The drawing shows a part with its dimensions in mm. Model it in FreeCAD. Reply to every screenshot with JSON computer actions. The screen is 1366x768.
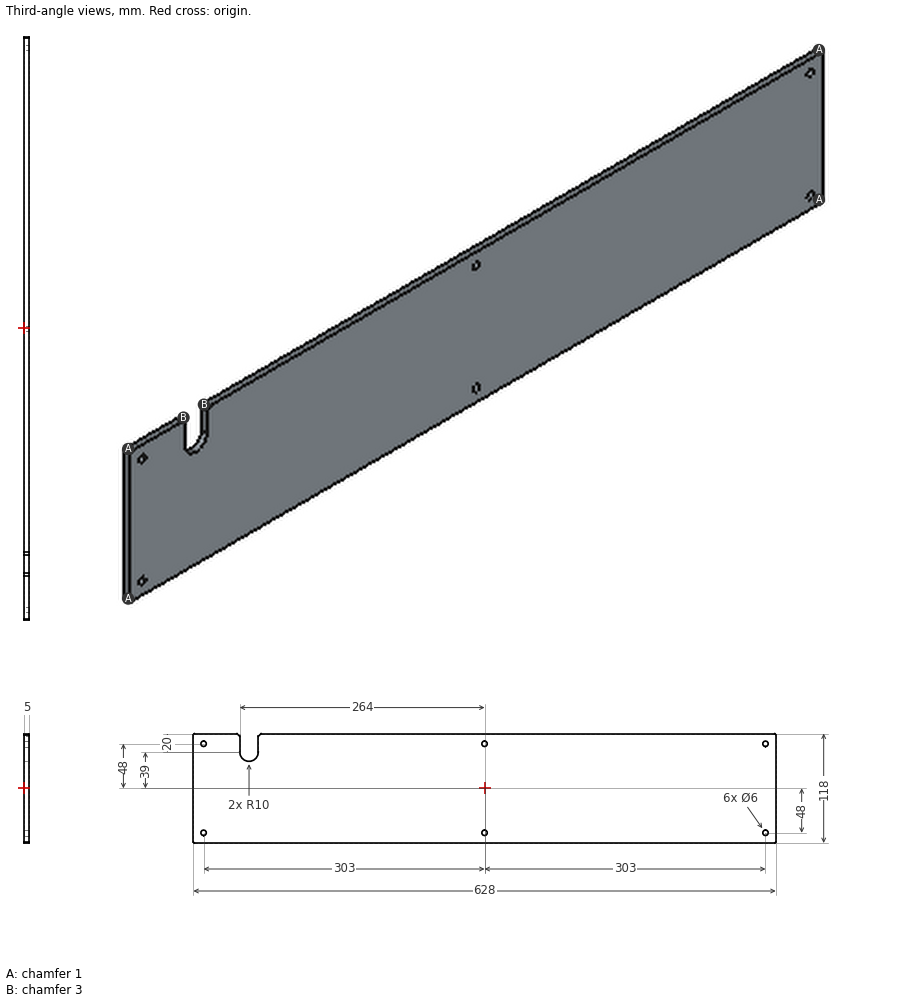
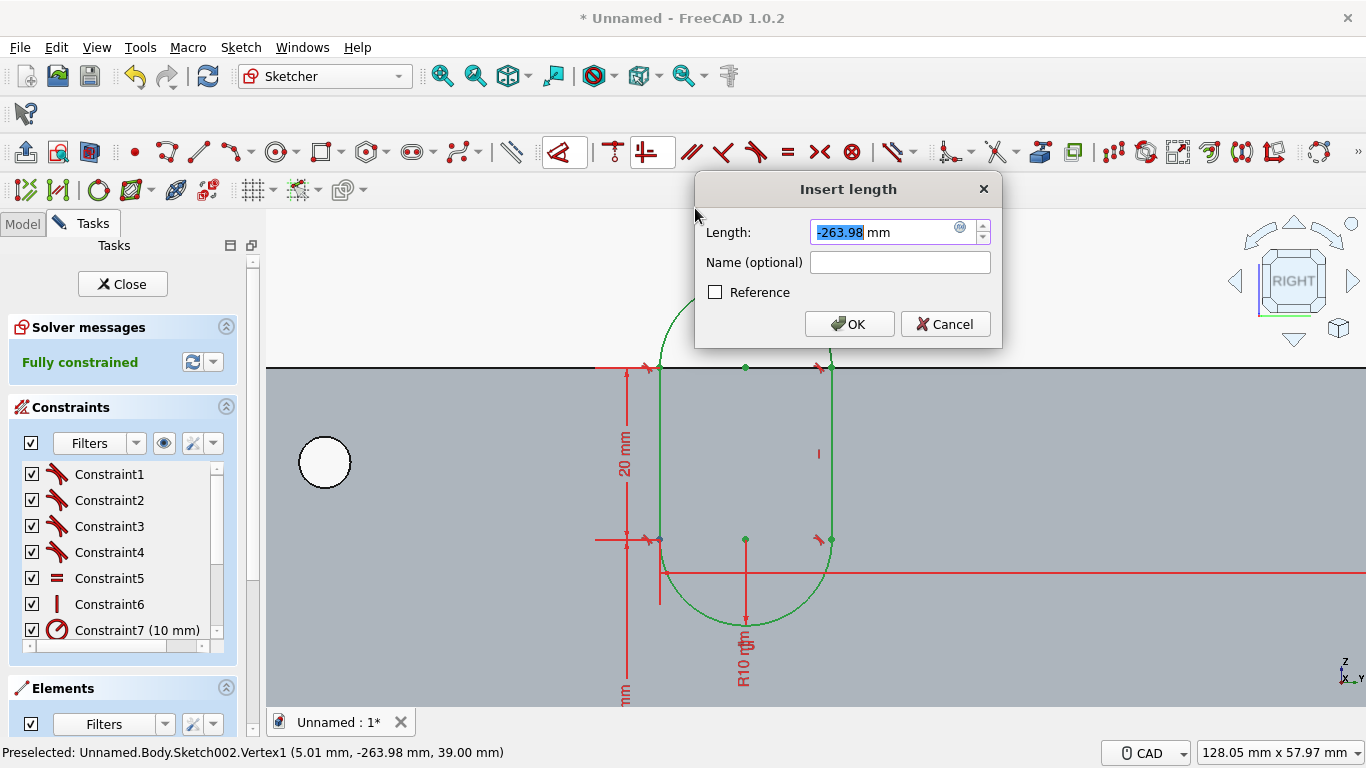
{"action": "type", "text": "-264"}
{"action": "key", "text": "Return"}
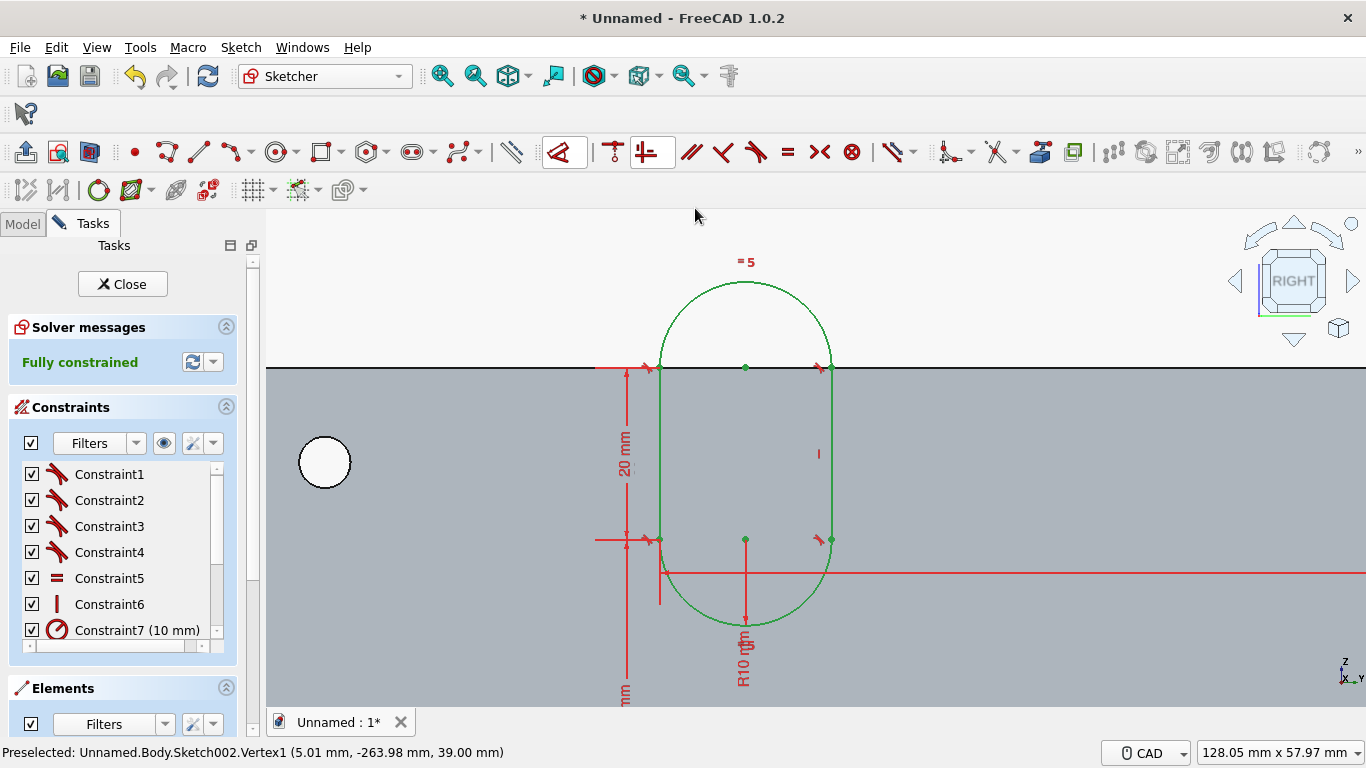
{"action": "left_click", "coordinate": [123, 284]}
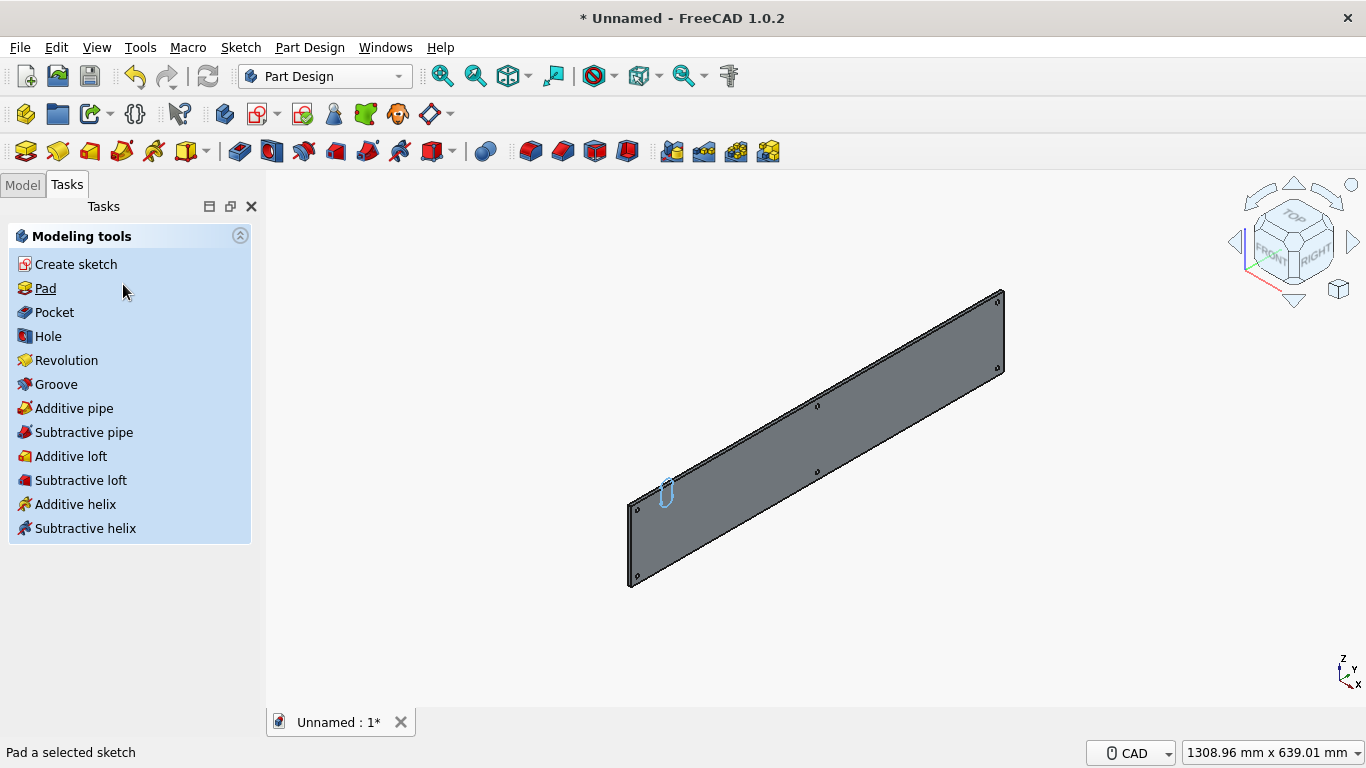
{"action": "left_click", "coordinate": [240, 152]}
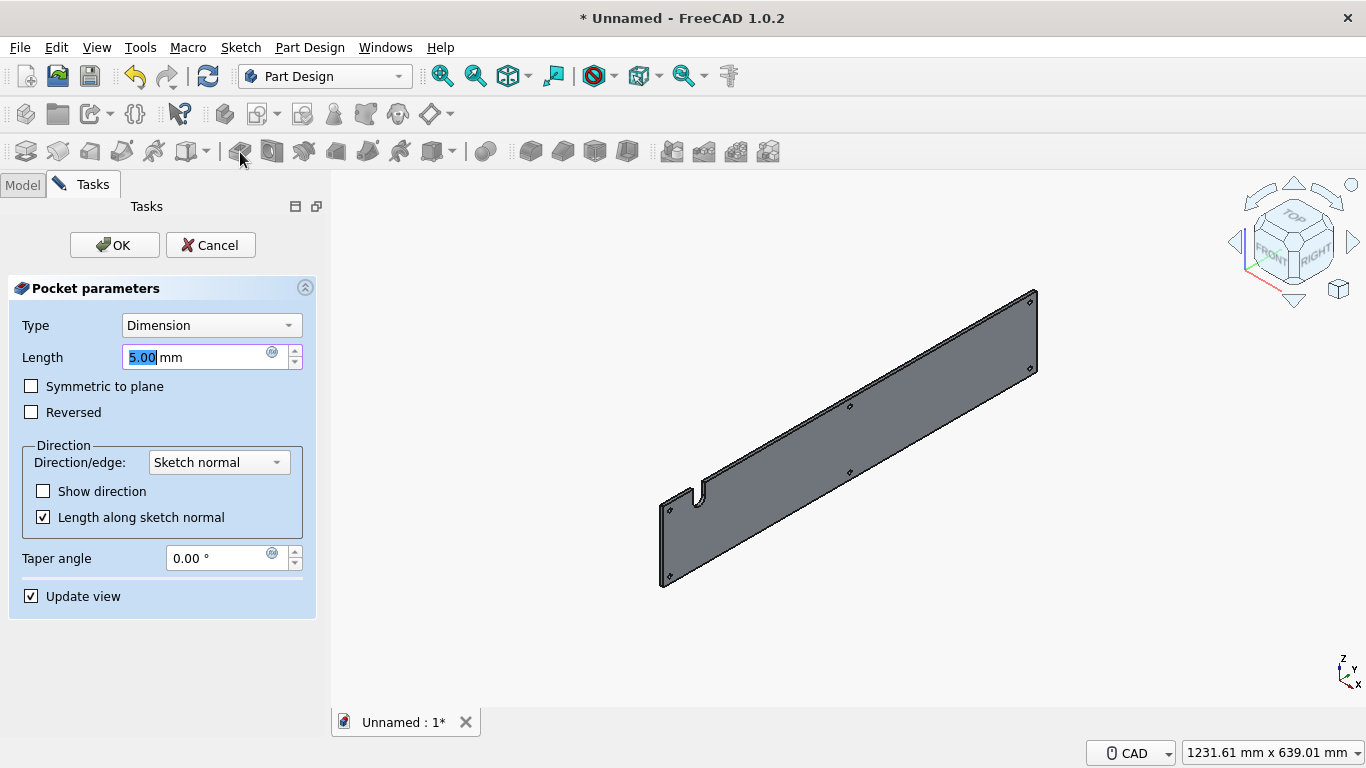
{"action": "left_click", "coordinate": [212, 326]}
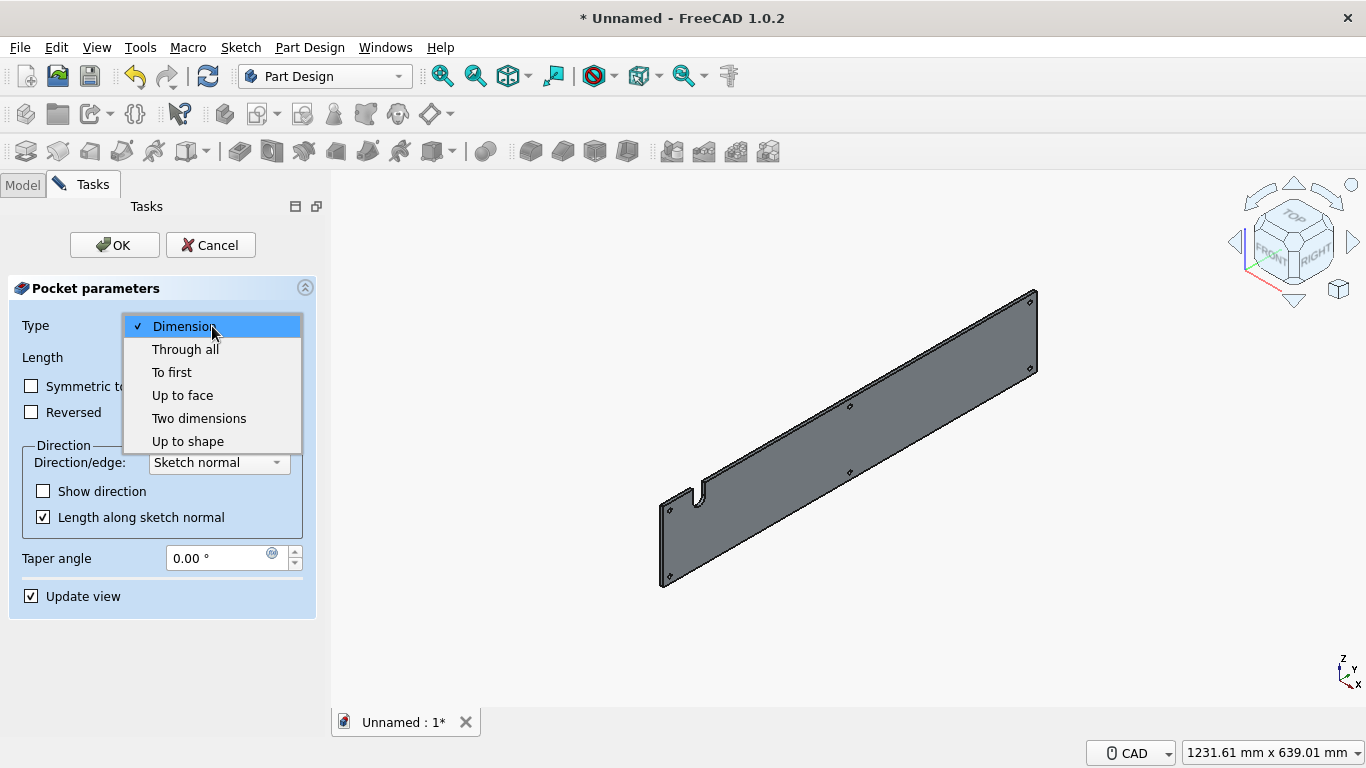
{"action": "left_click", "coordinate": [212, 350]}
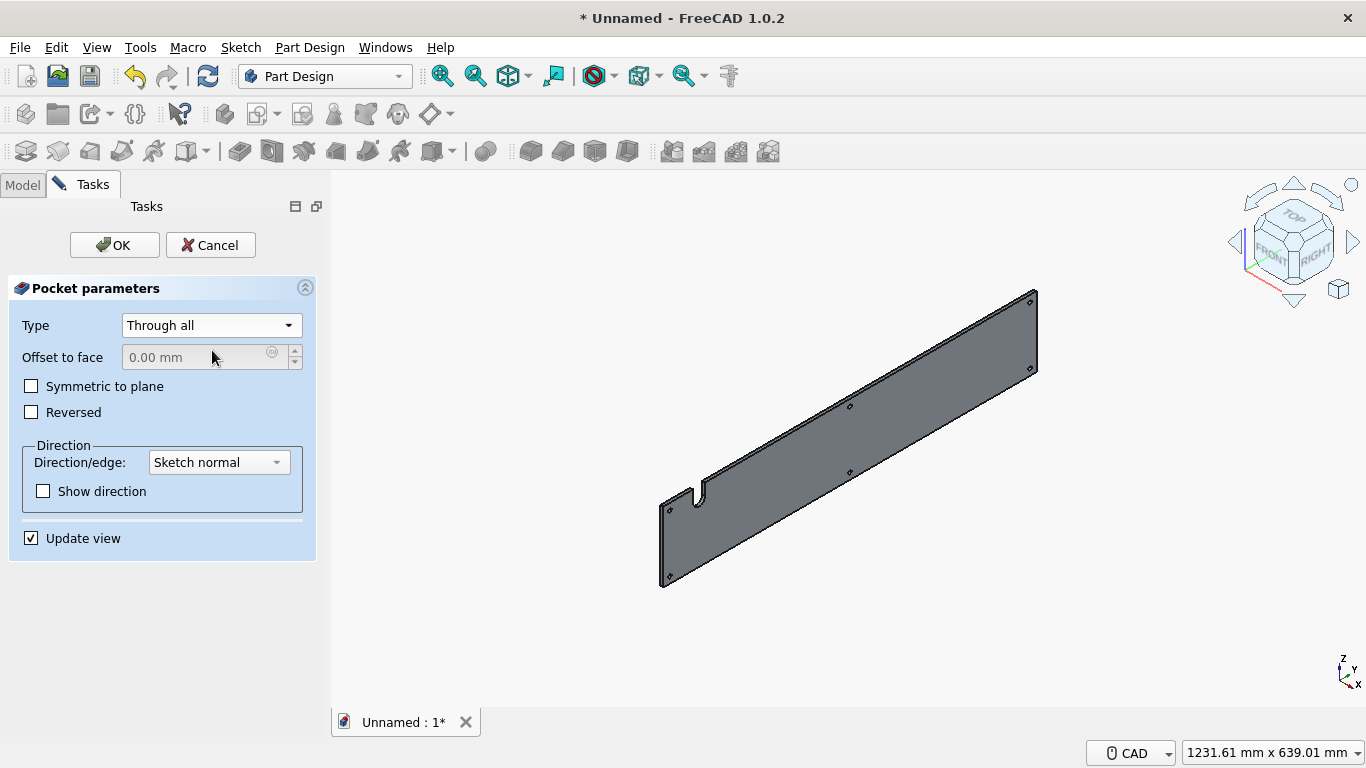
{"action": "left_click", "coordinate": [115, 245]}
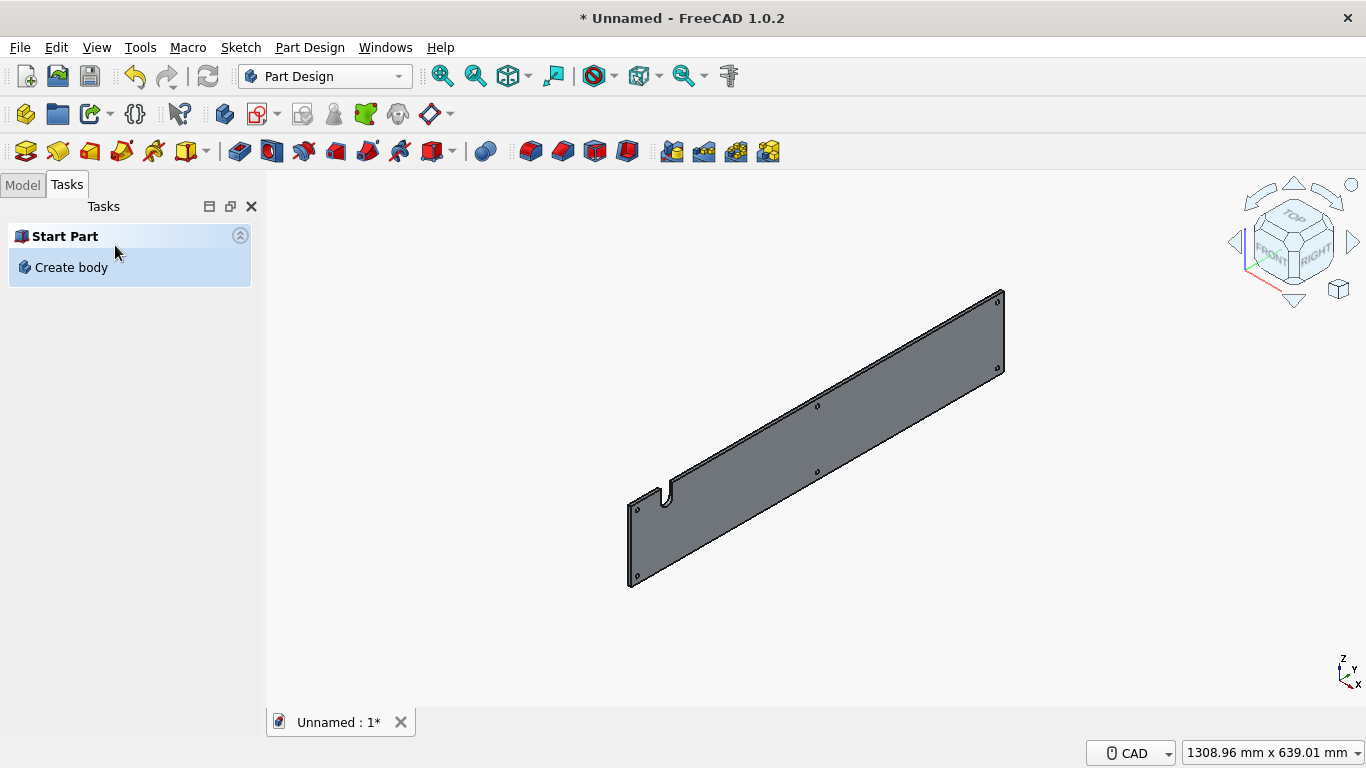
{"action": "scroll", "coordinate": [659, 488], "scroll_direction": "up", "scroll_amount": 12}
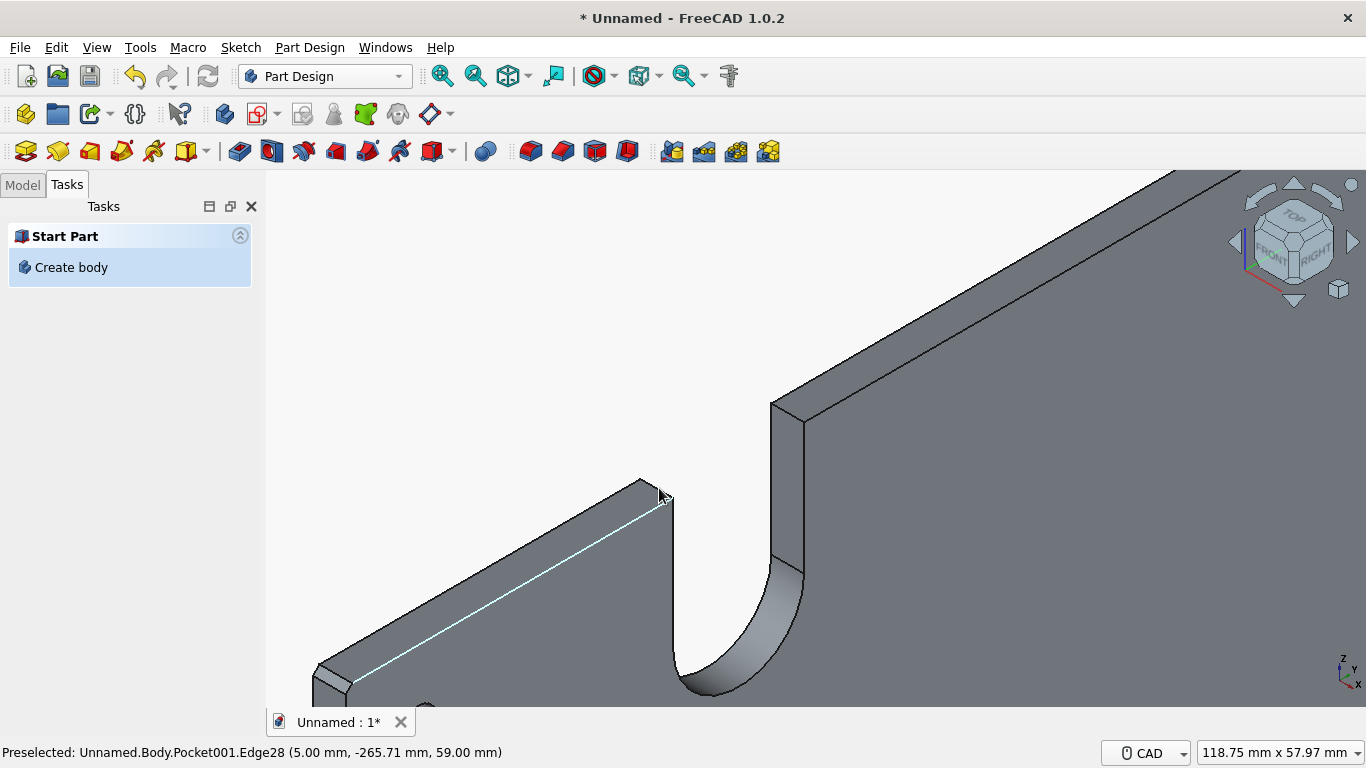
{"action": "left_click", "coordinate": [788, 412]}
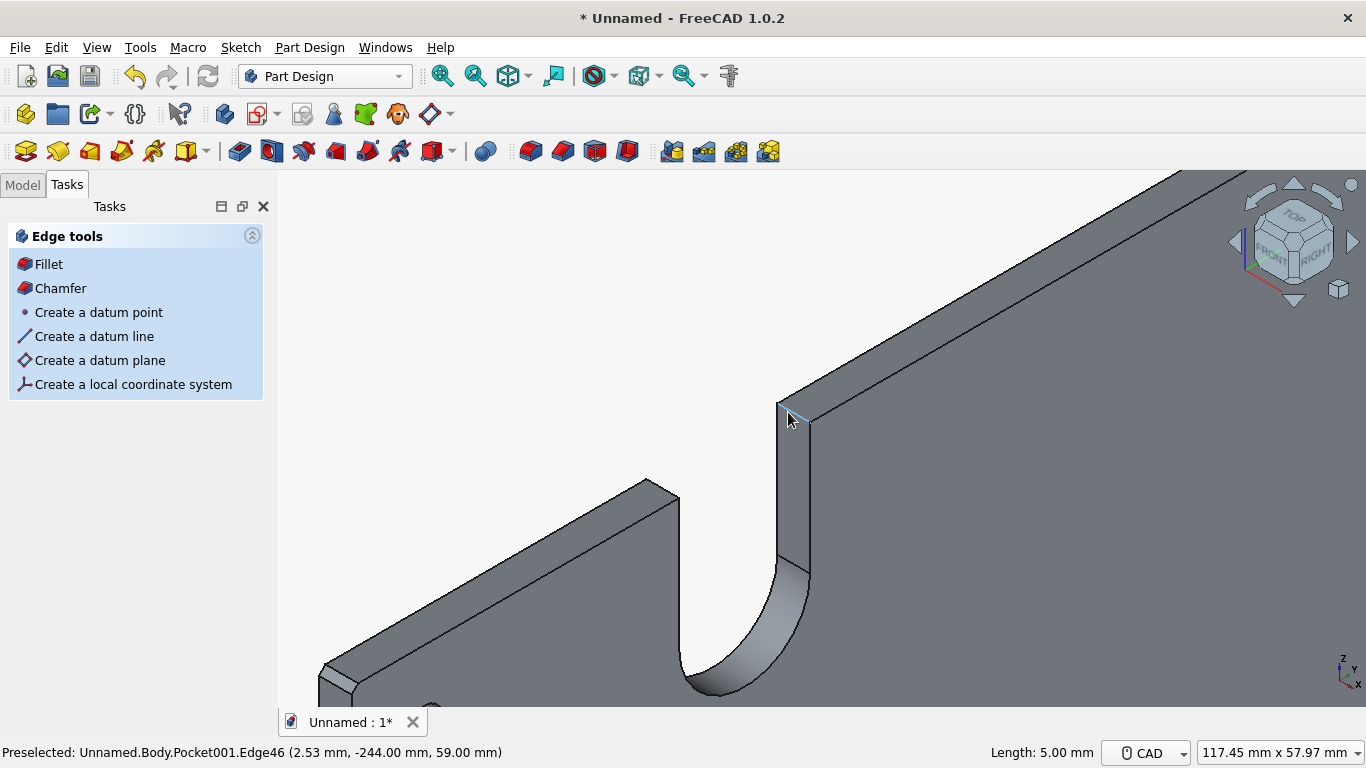
{"action": "left_click", "coordinate": [444, 76]}